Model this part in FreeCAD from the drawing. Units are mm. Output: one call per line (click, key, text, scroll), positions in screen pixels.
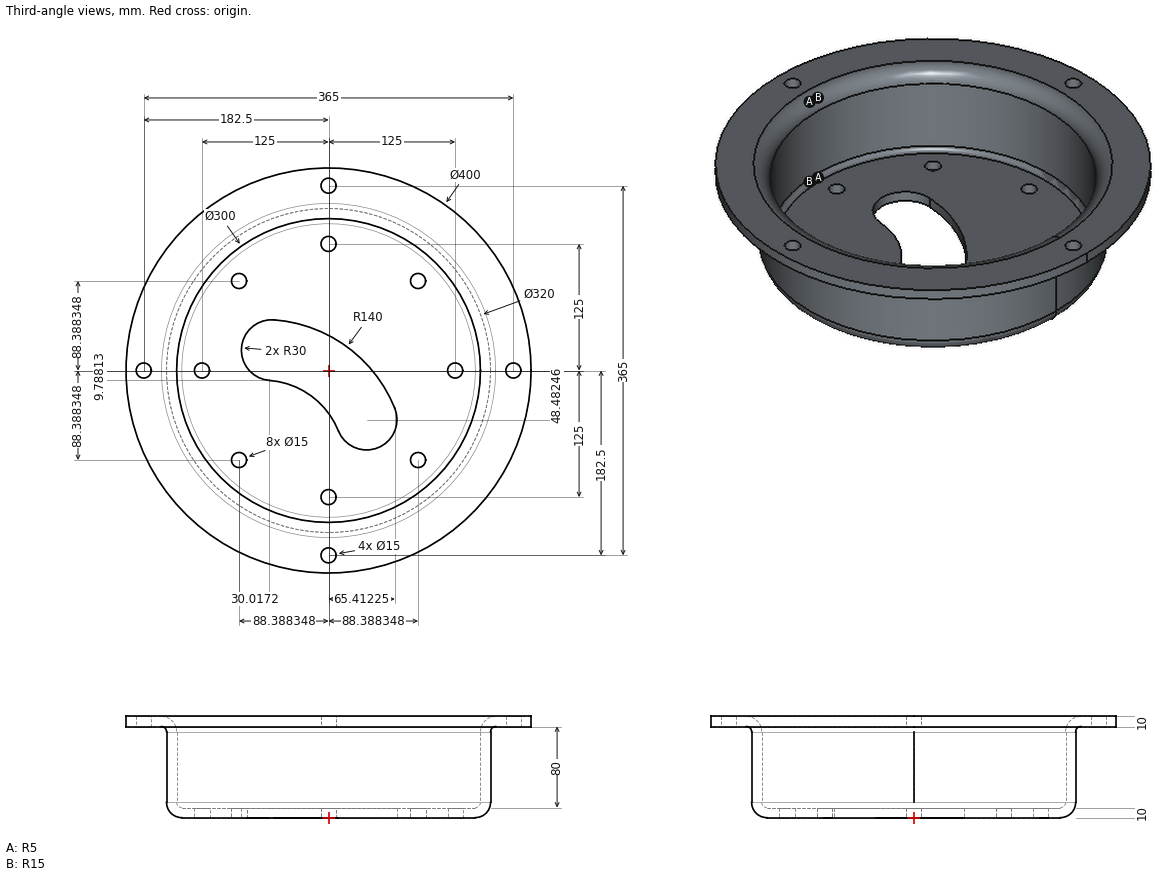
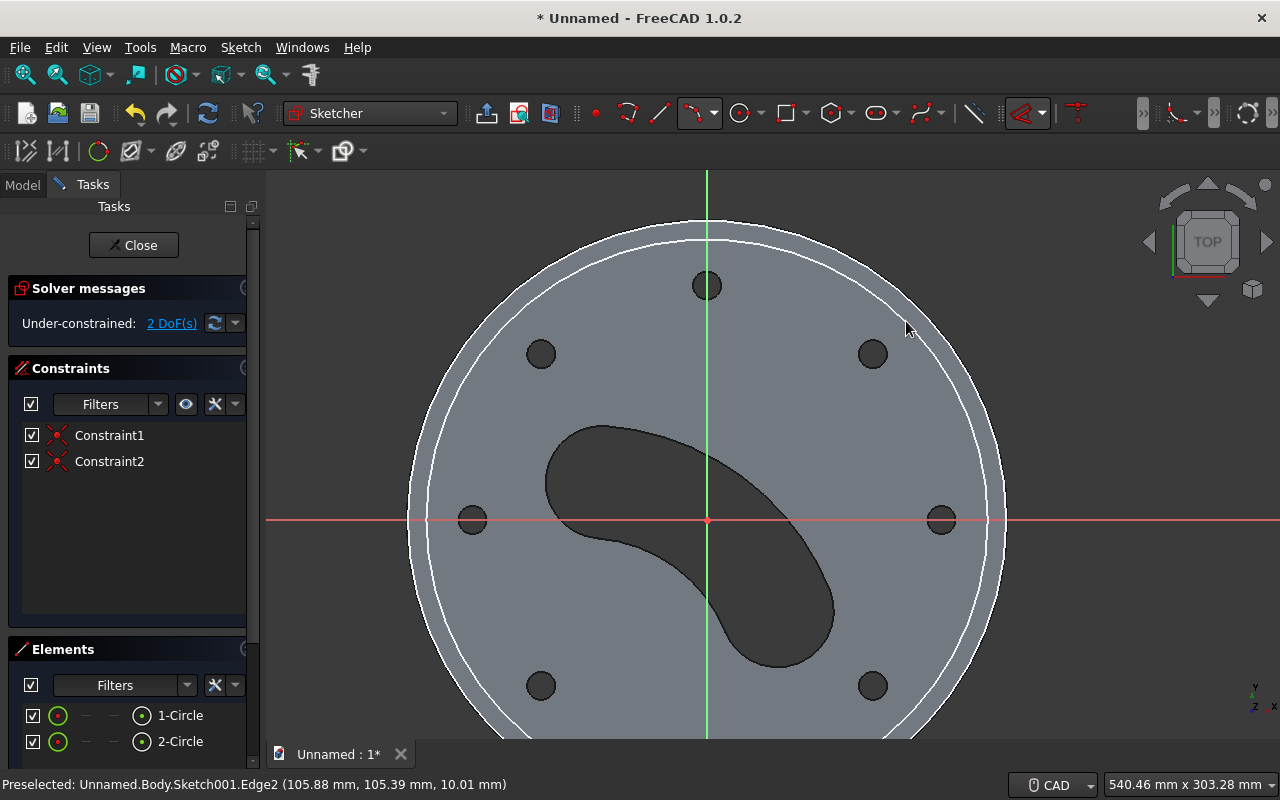
click(918, 308)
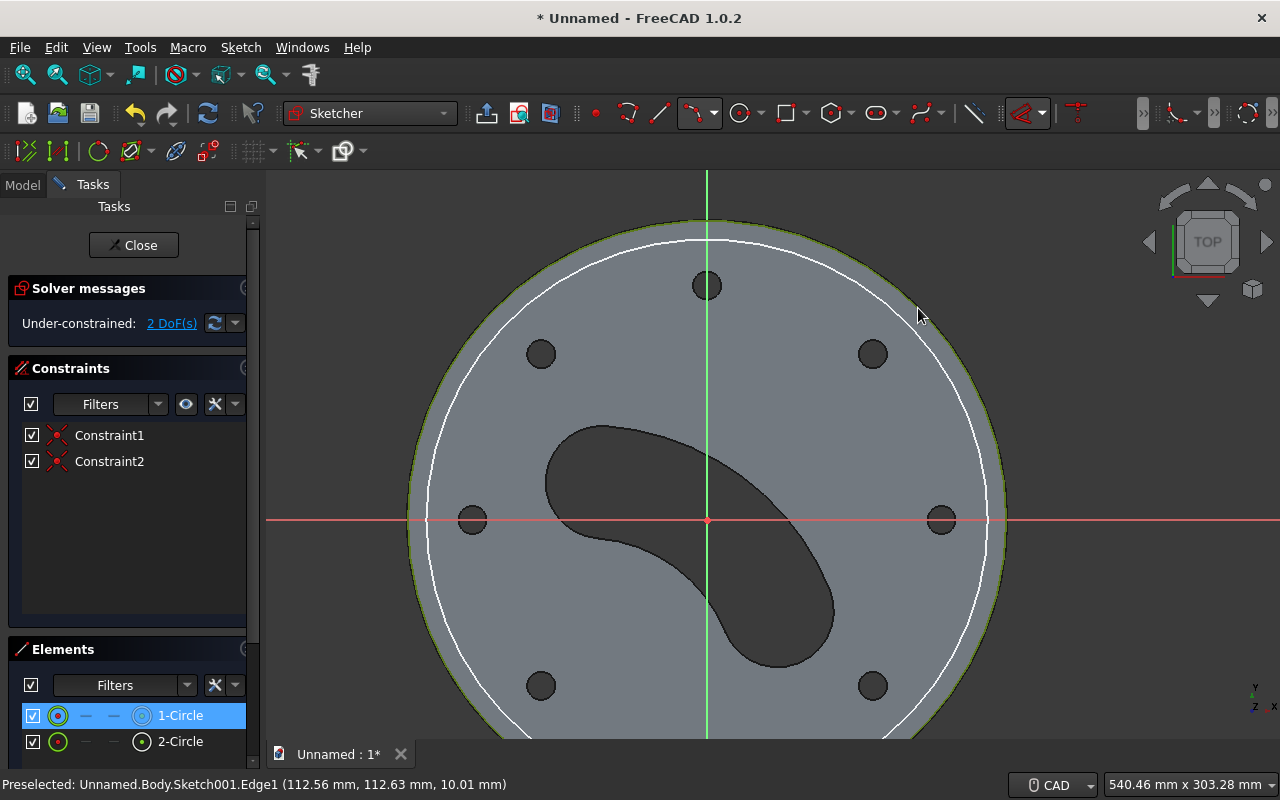
click(1044, 114)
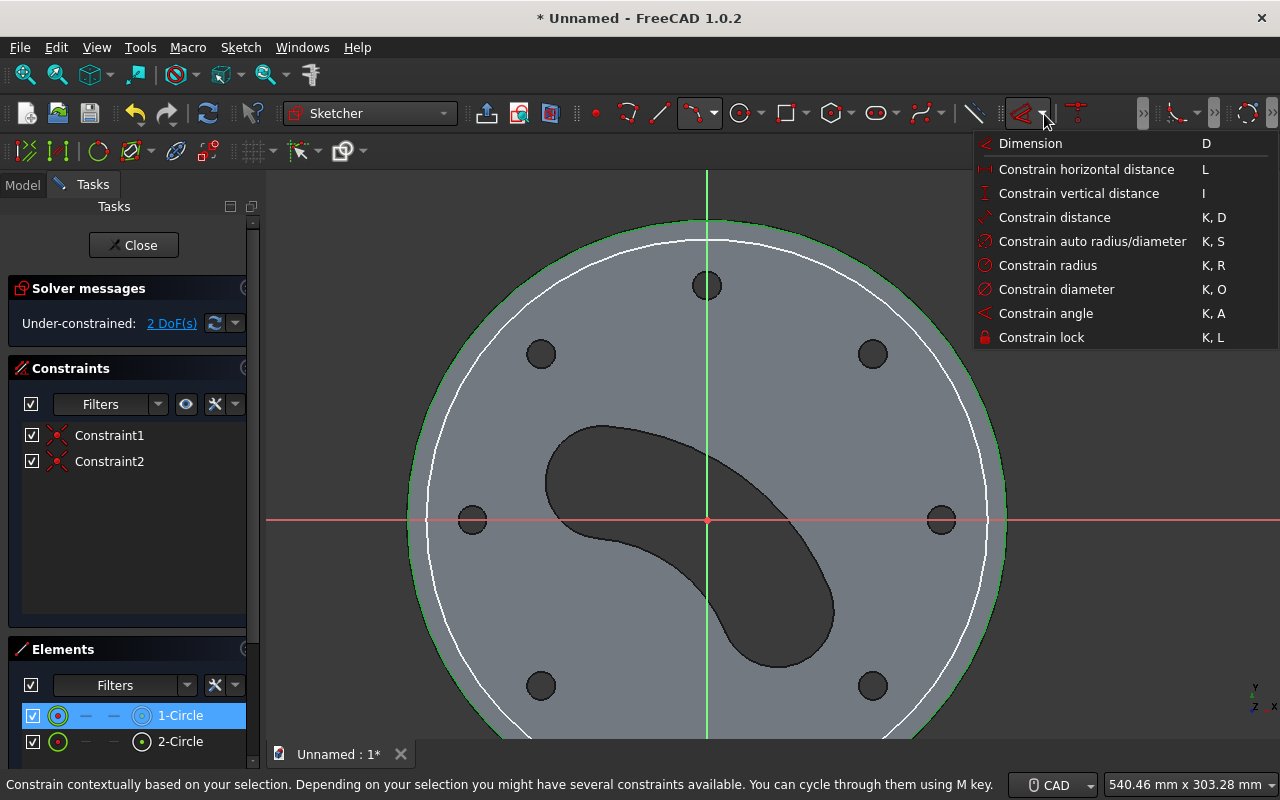
click(1126, 289)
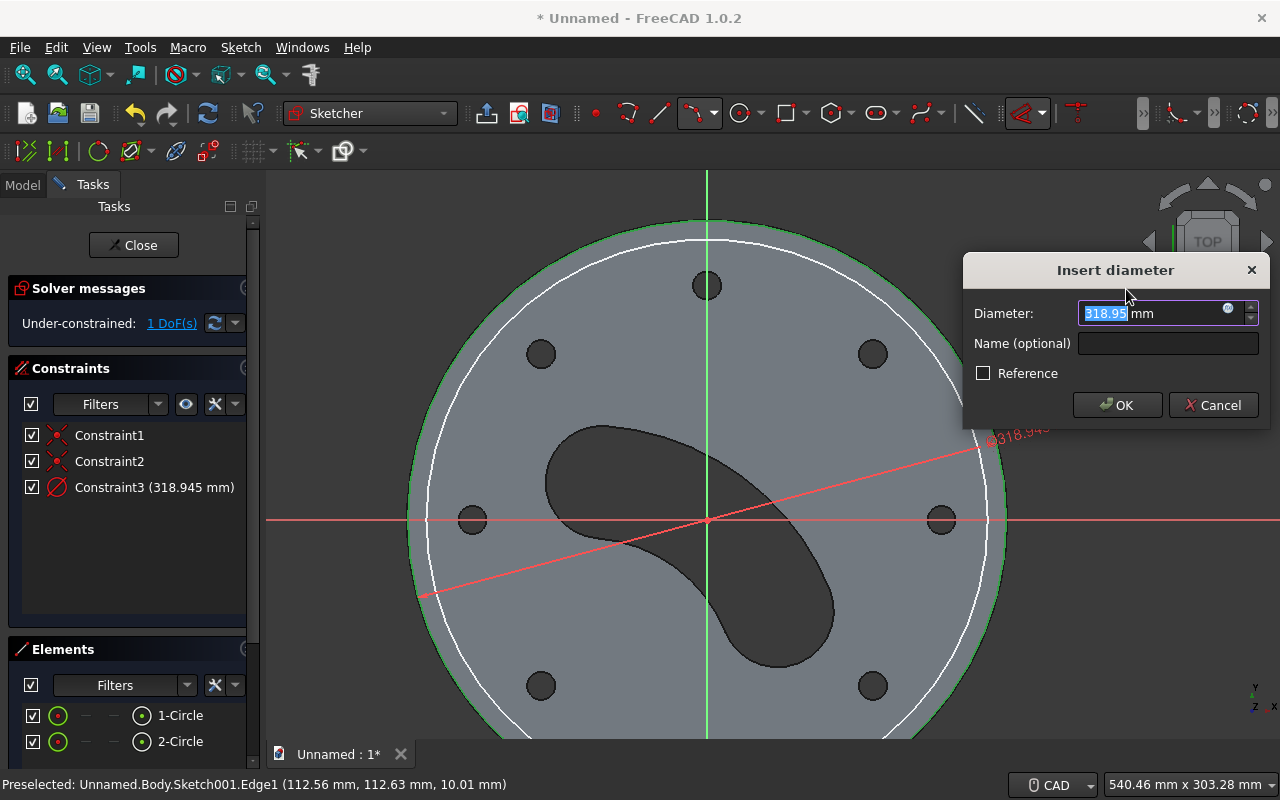
text(320)
key(Return)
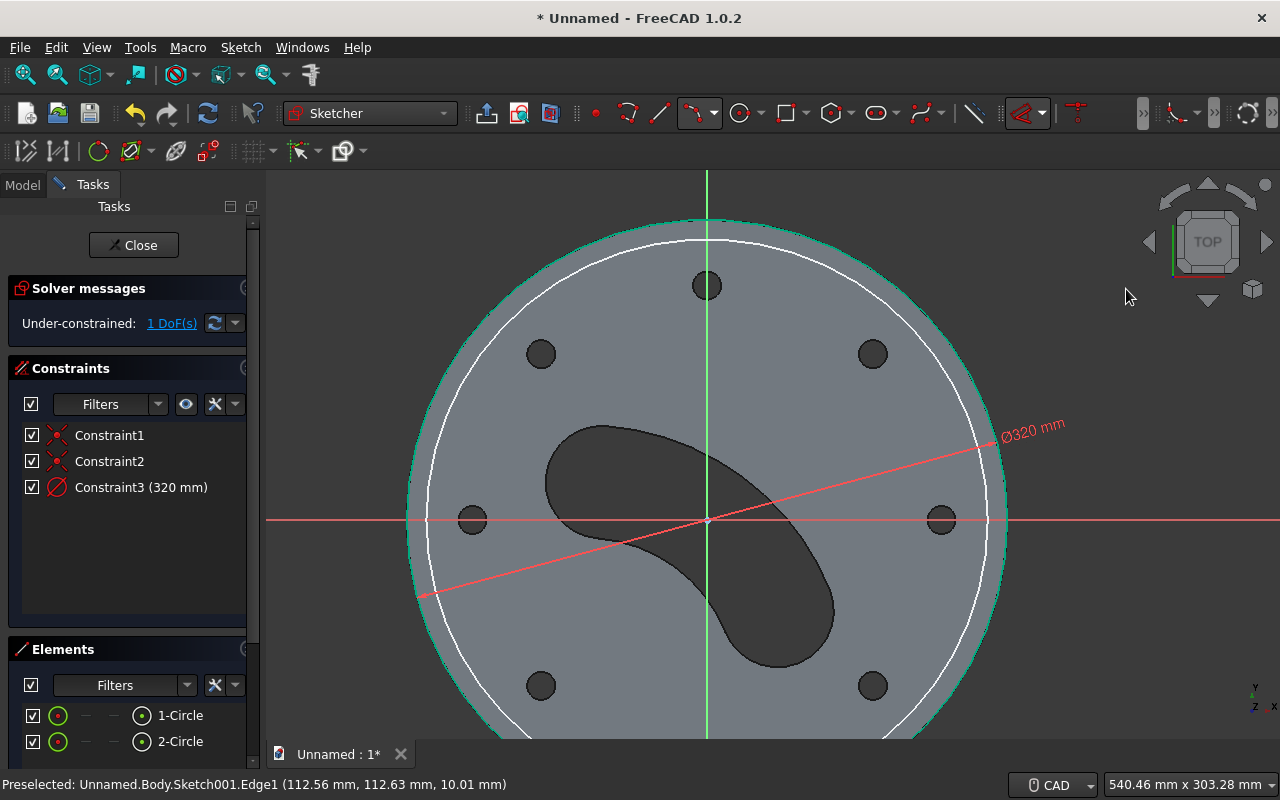
click(905, 321)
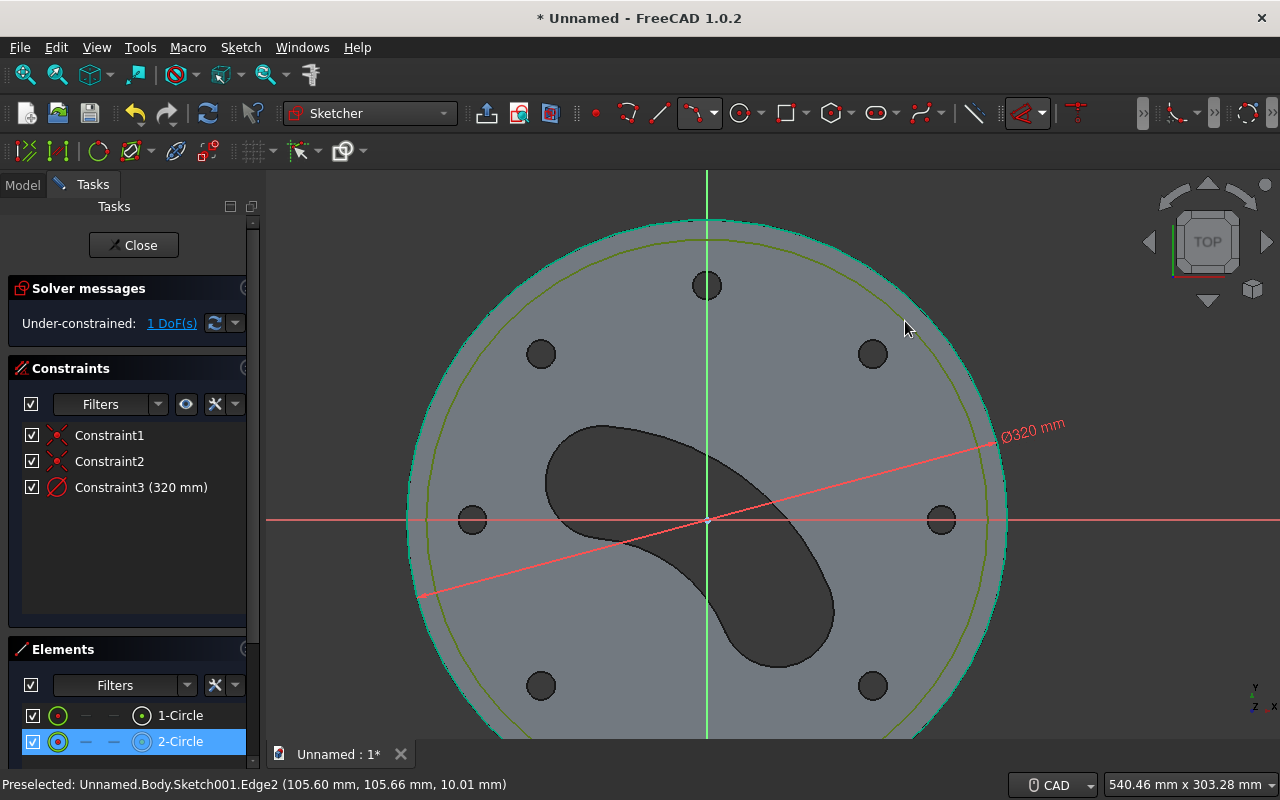
key(k)
key(o)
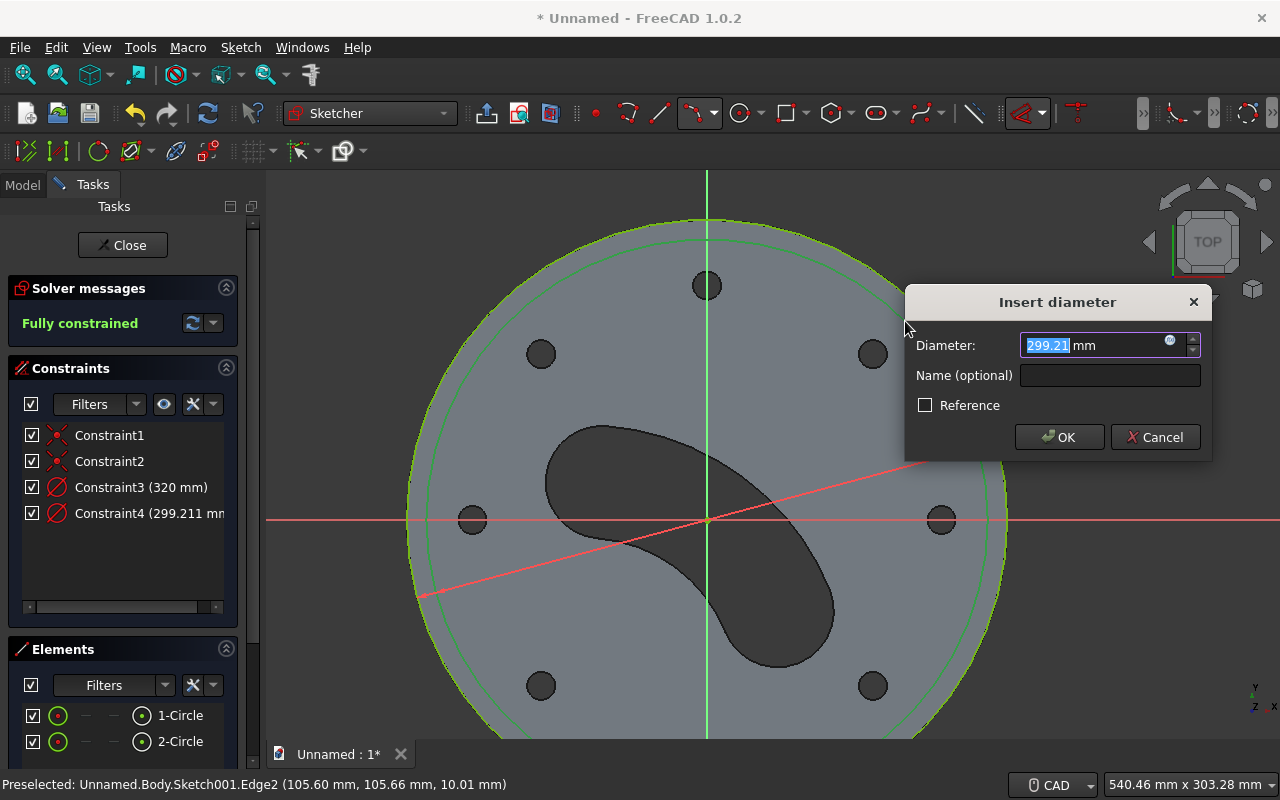
text(300)
key(Return)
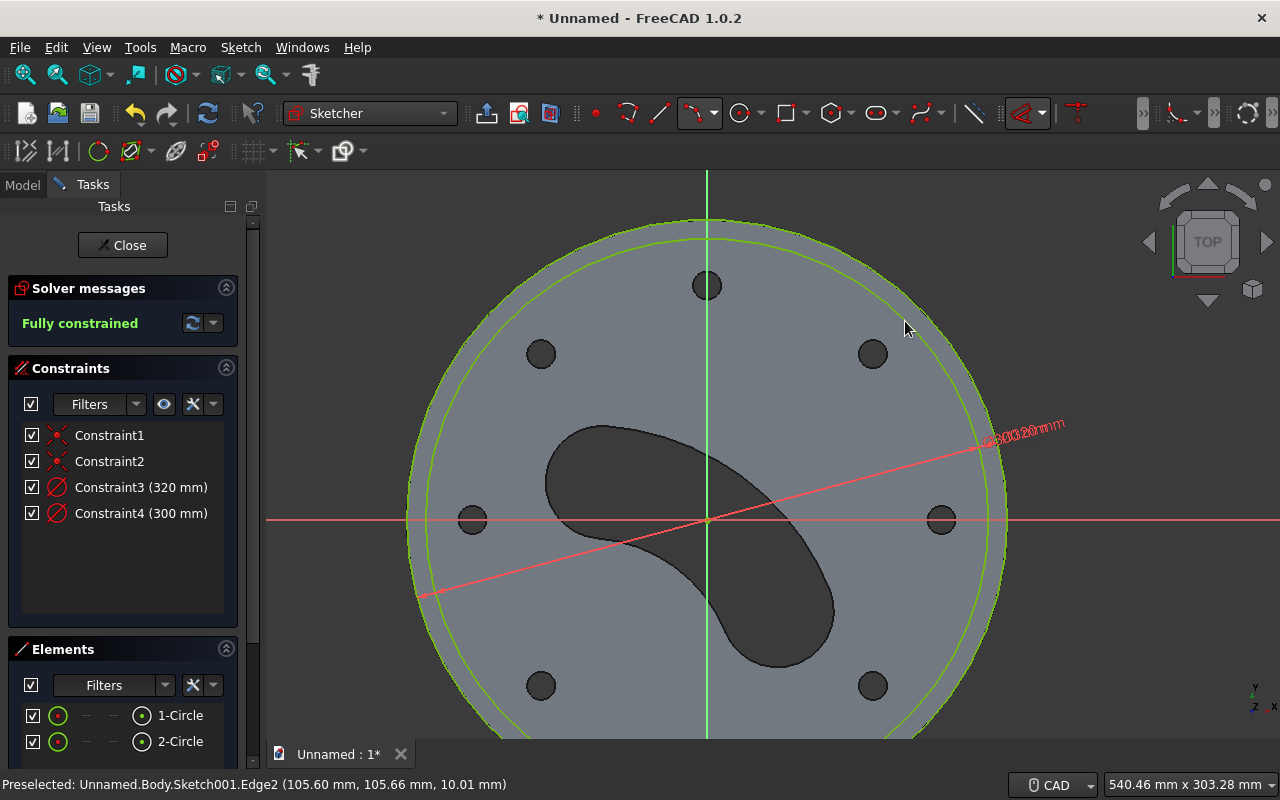
click(123, 245)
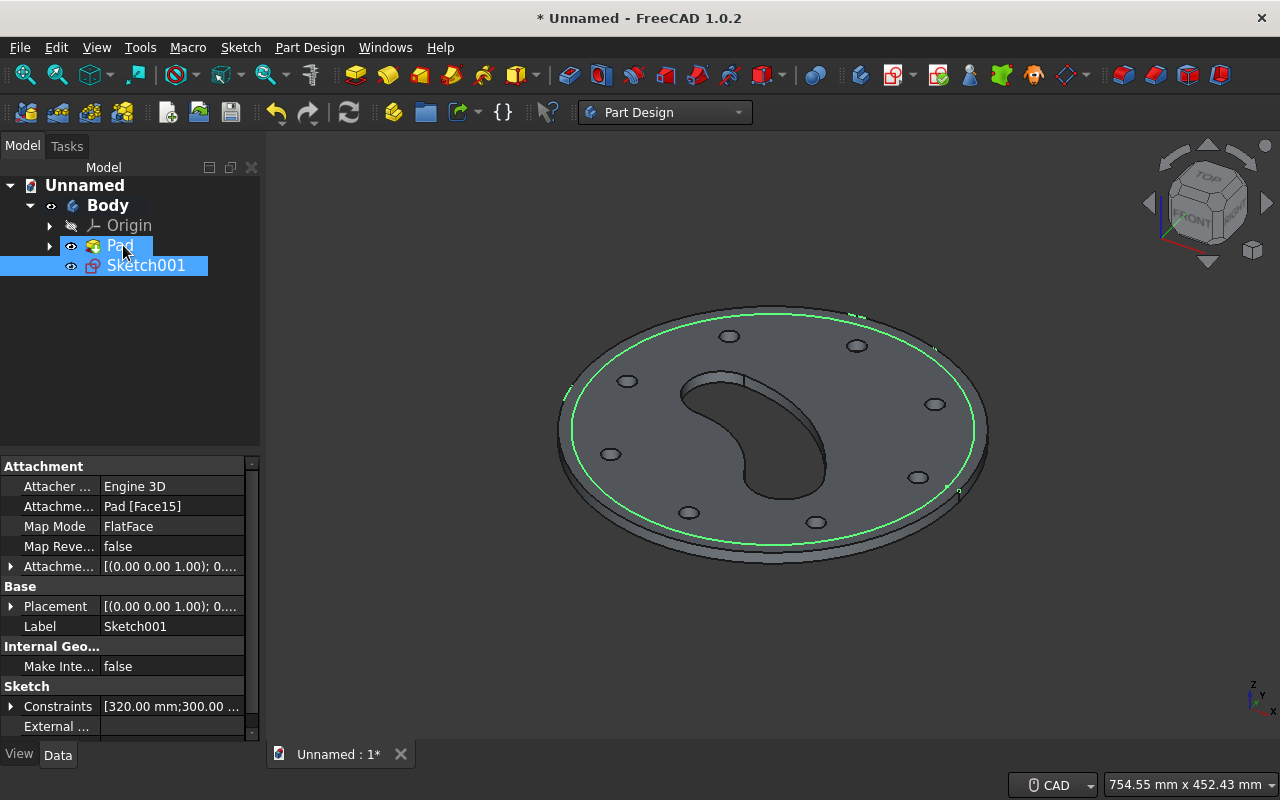
click(356, 76)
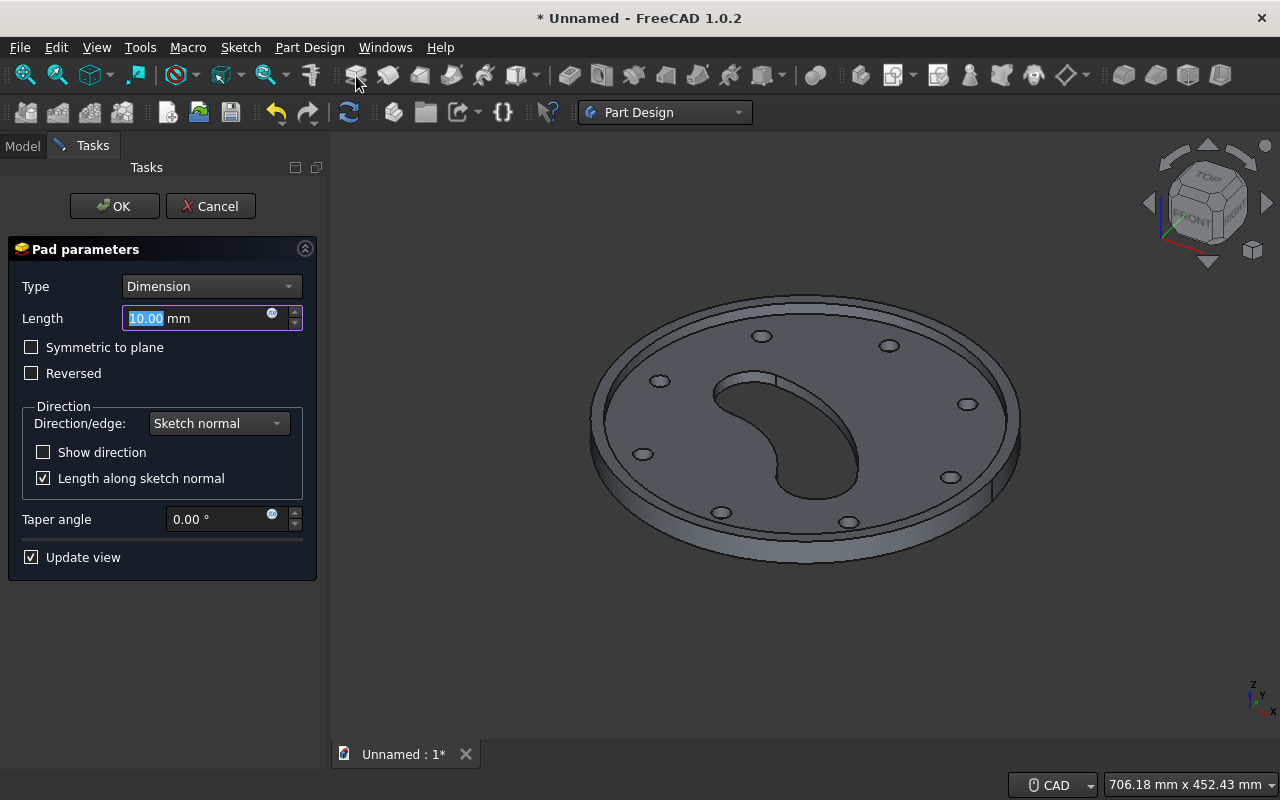
text(80)
key(Tab)